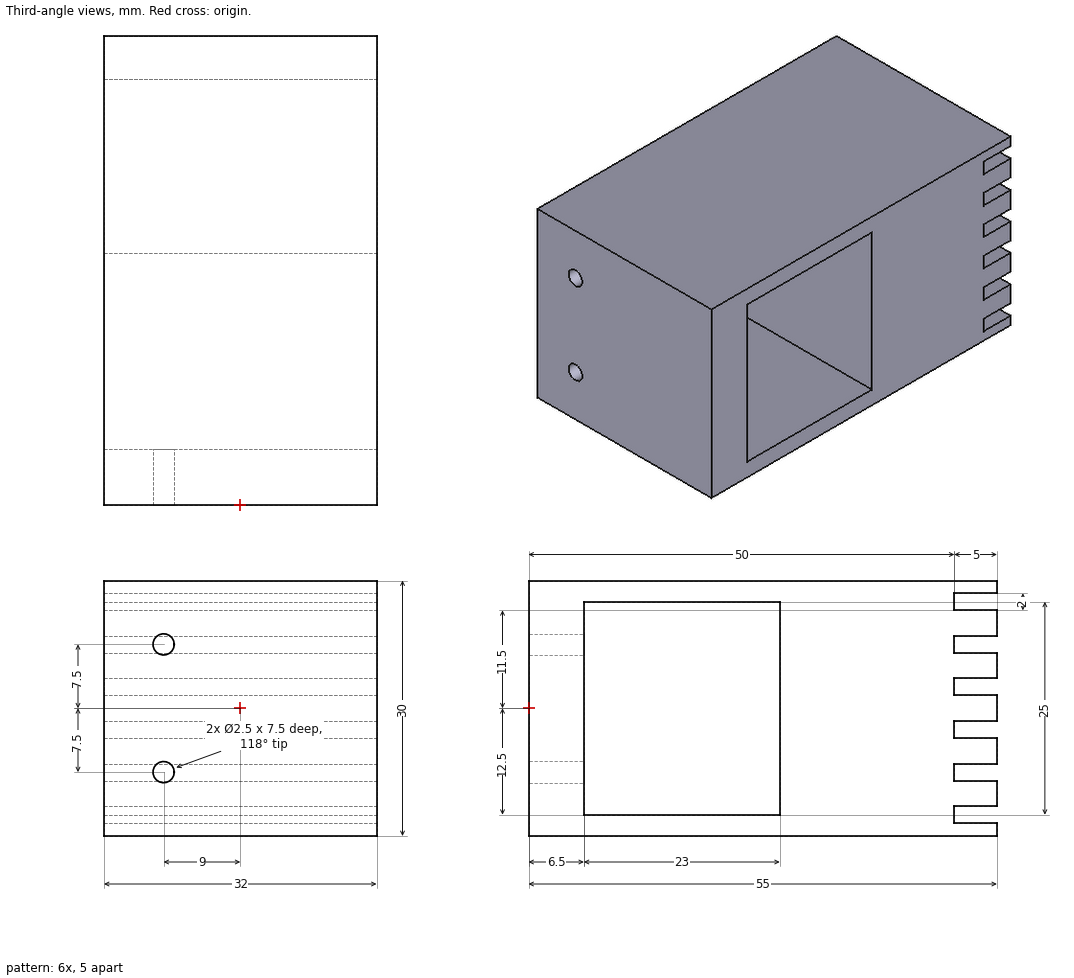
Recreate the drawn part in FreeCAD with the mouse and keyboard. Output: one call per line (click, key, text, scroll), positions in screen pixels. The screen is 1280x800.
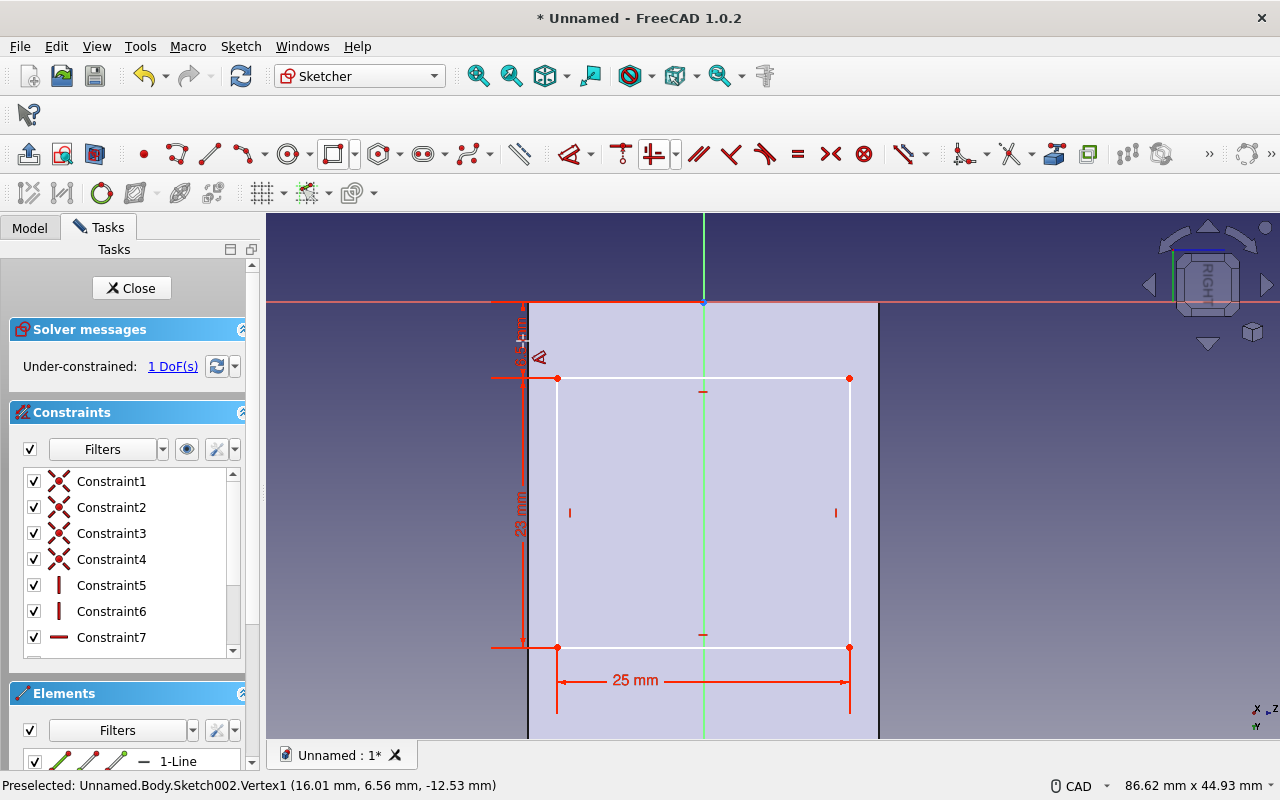
click(557, 378)
click(630, 268)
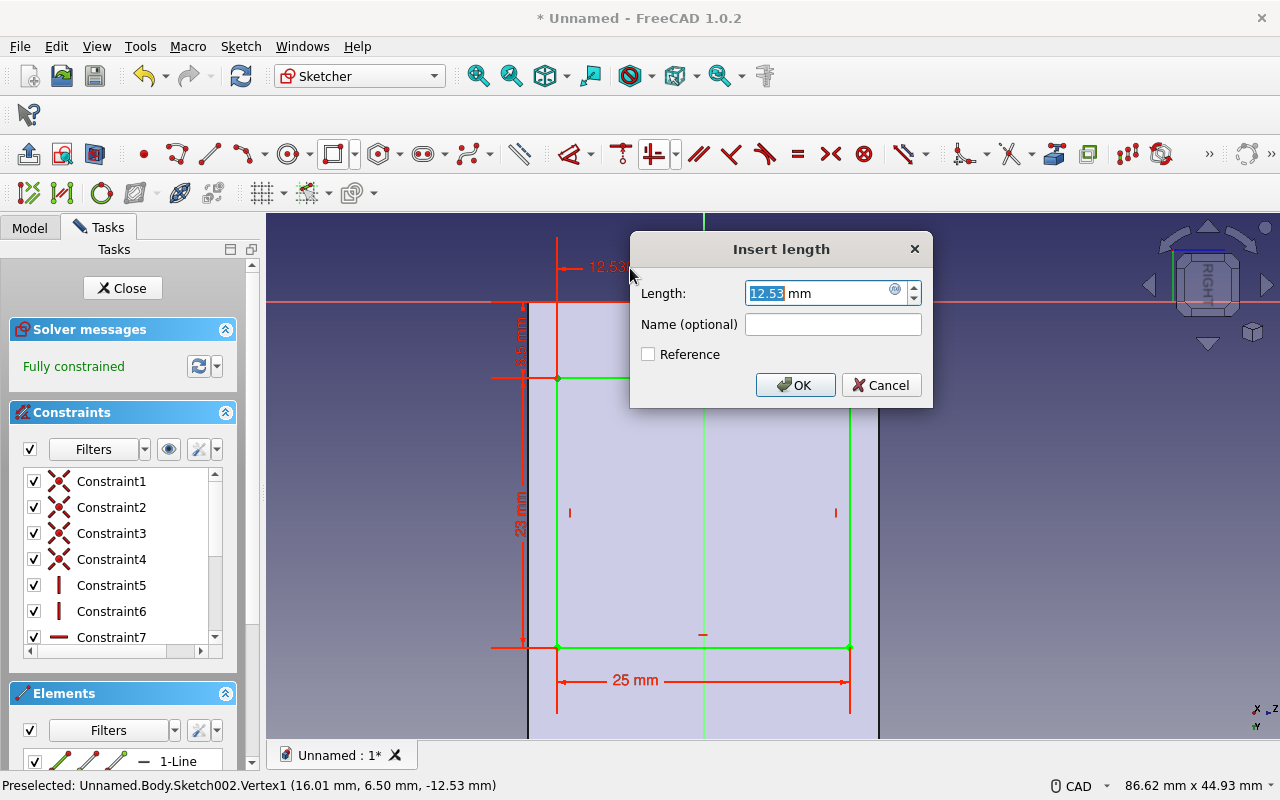
text(12.5)
key(Return)
key(Escape)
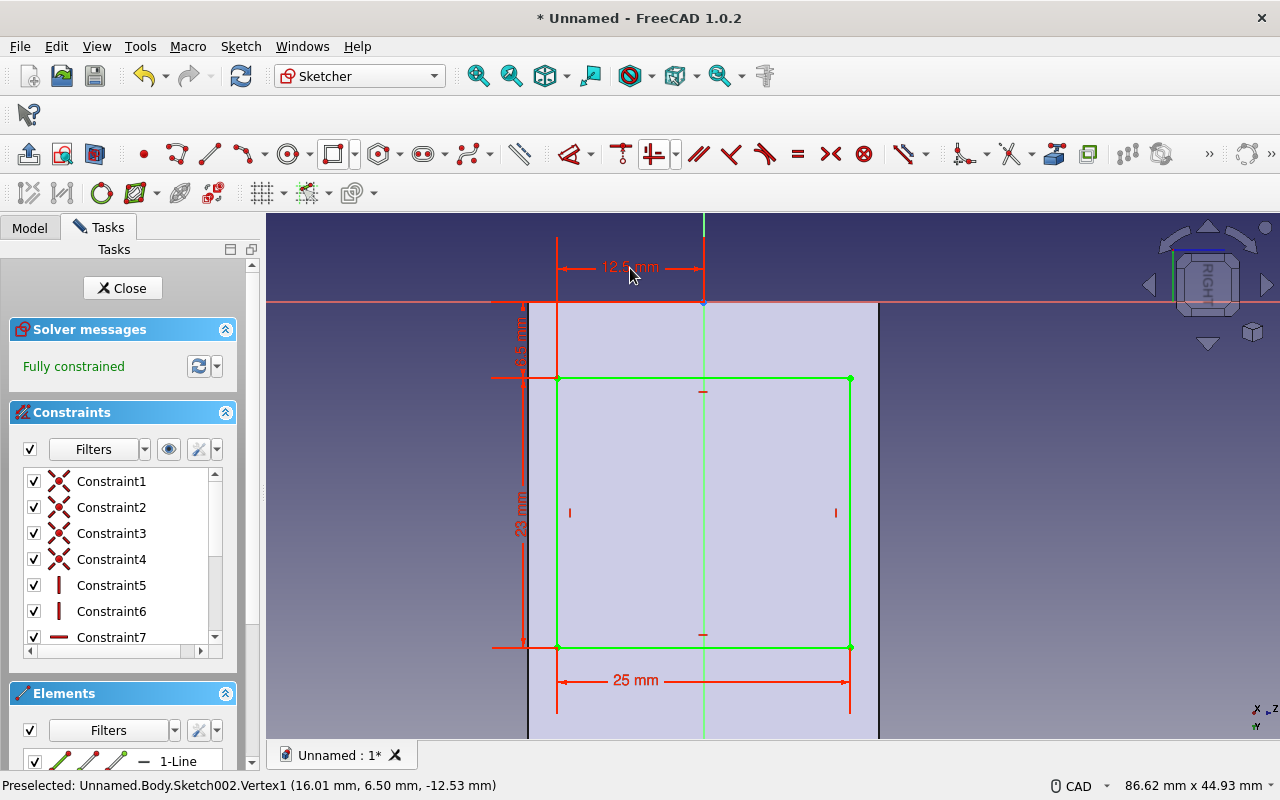
click(123, 288)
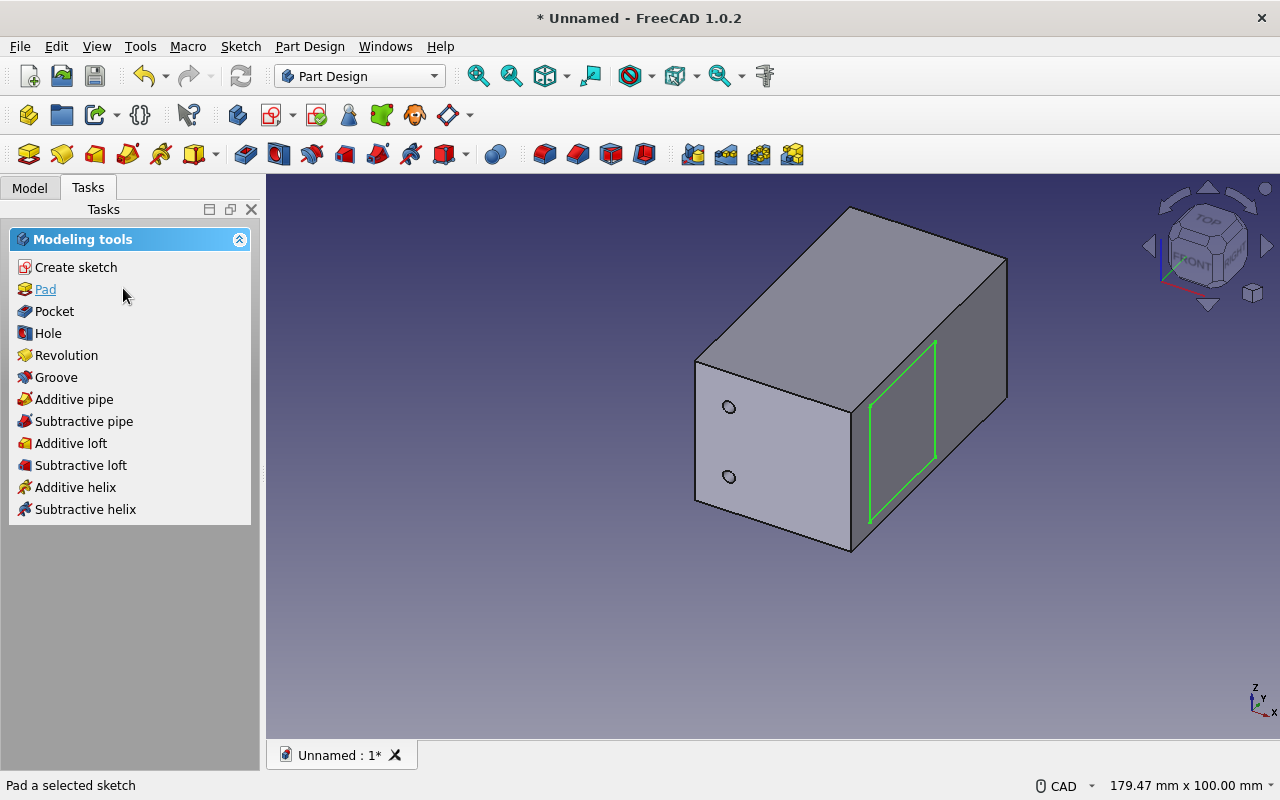
click(246, 154)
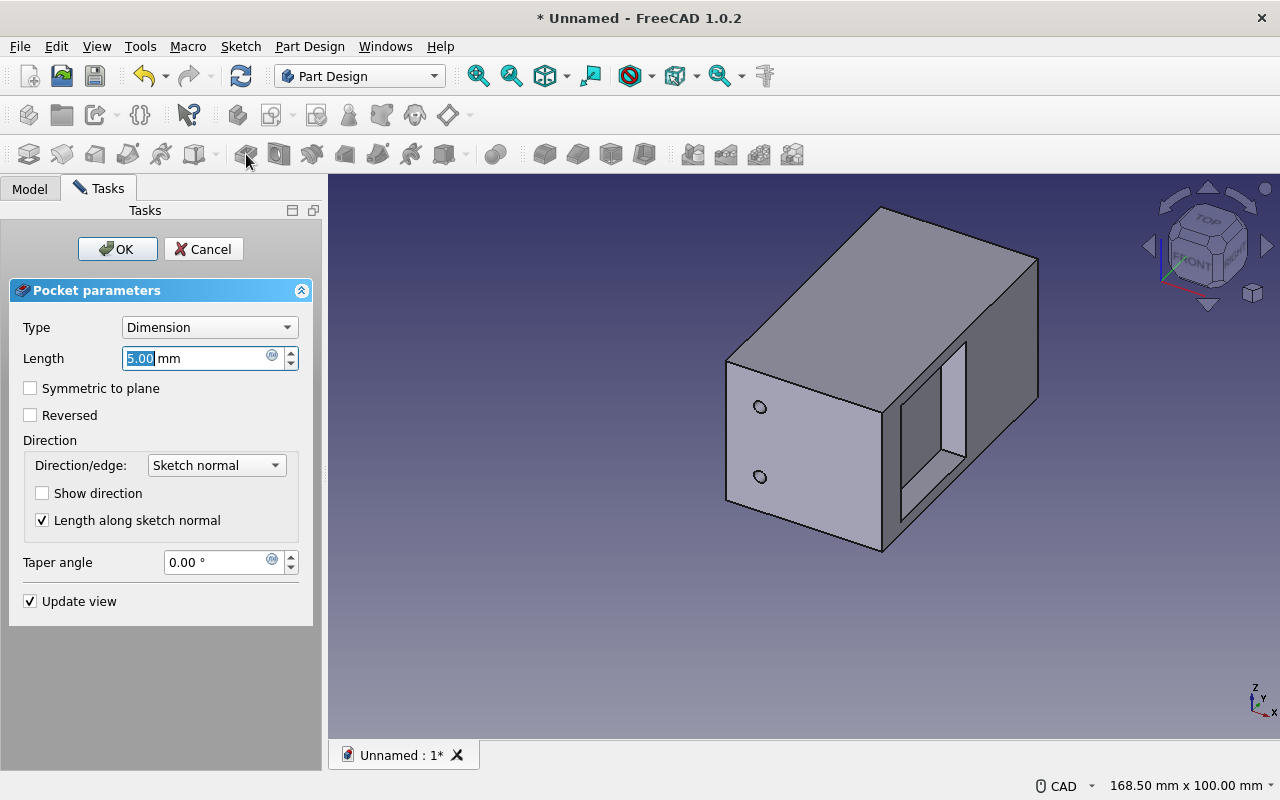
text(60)
key(Tab)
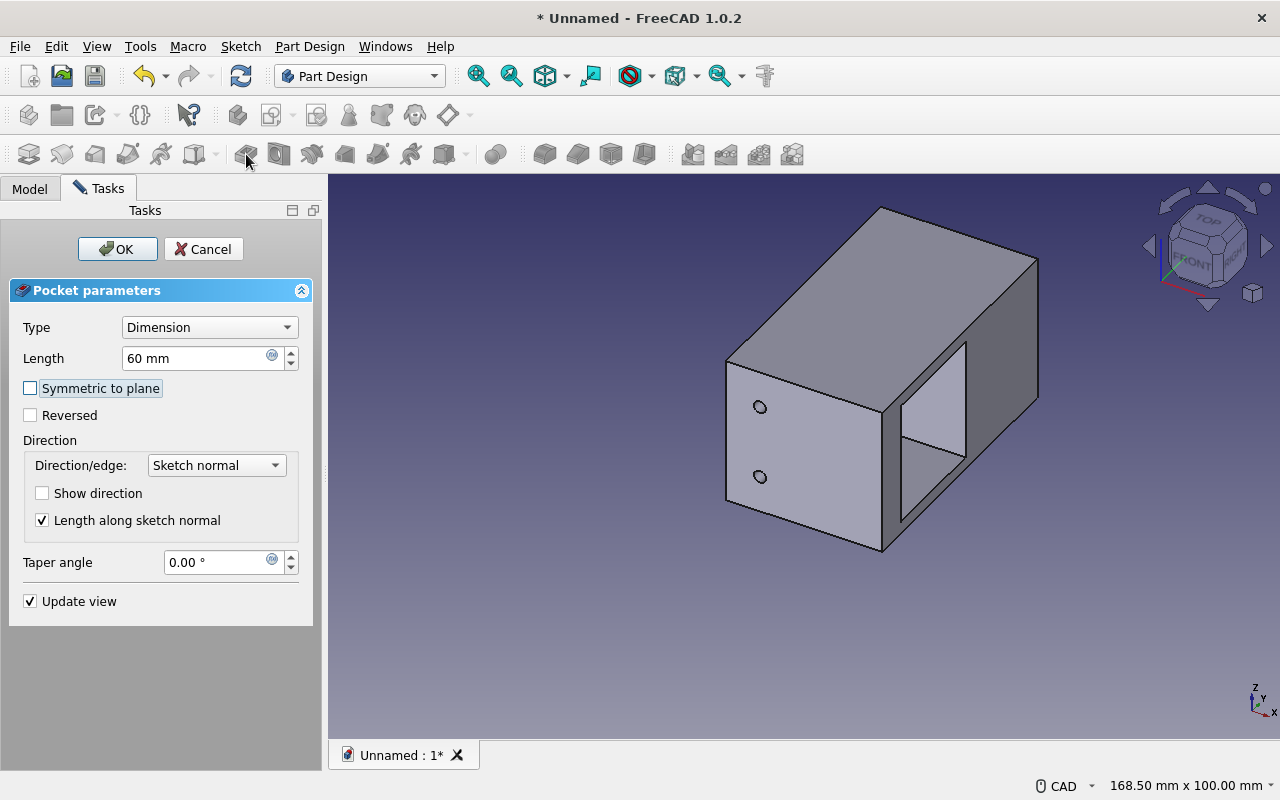
click(118, 249)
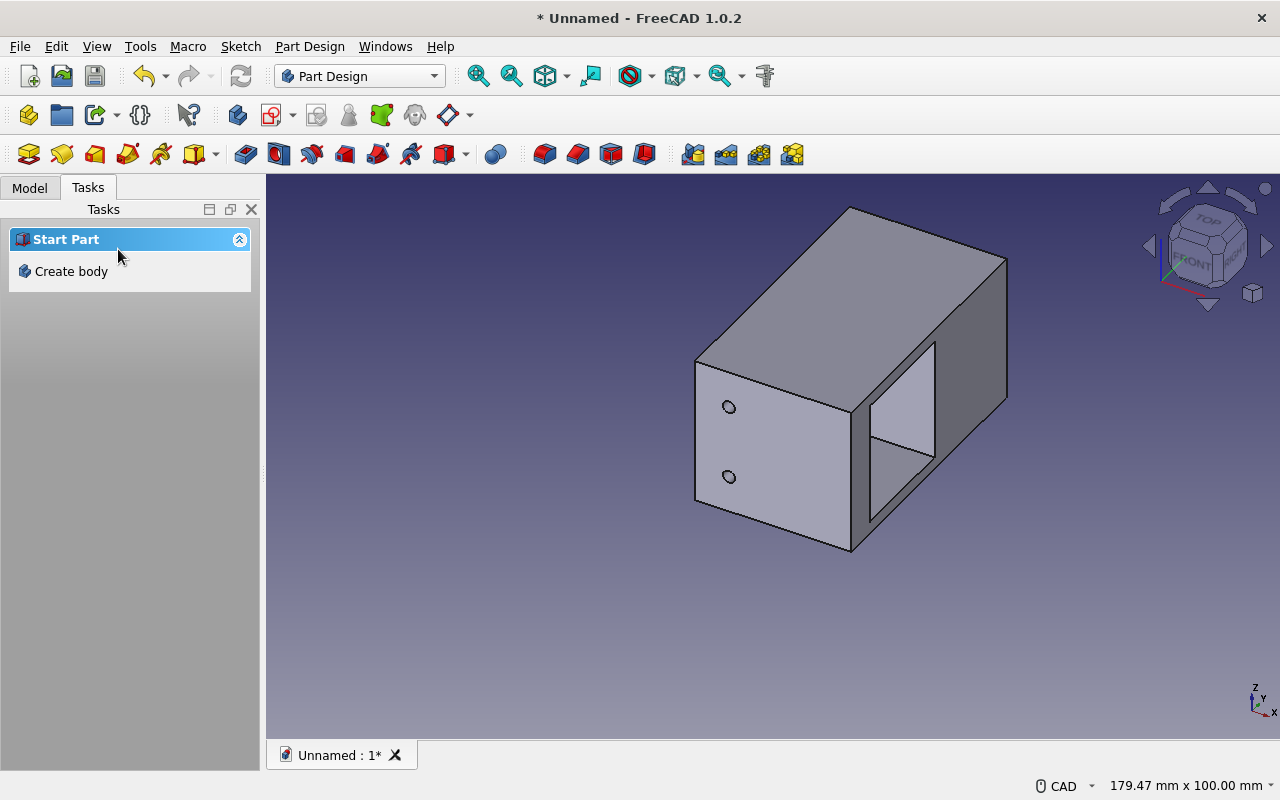
click(973, 360)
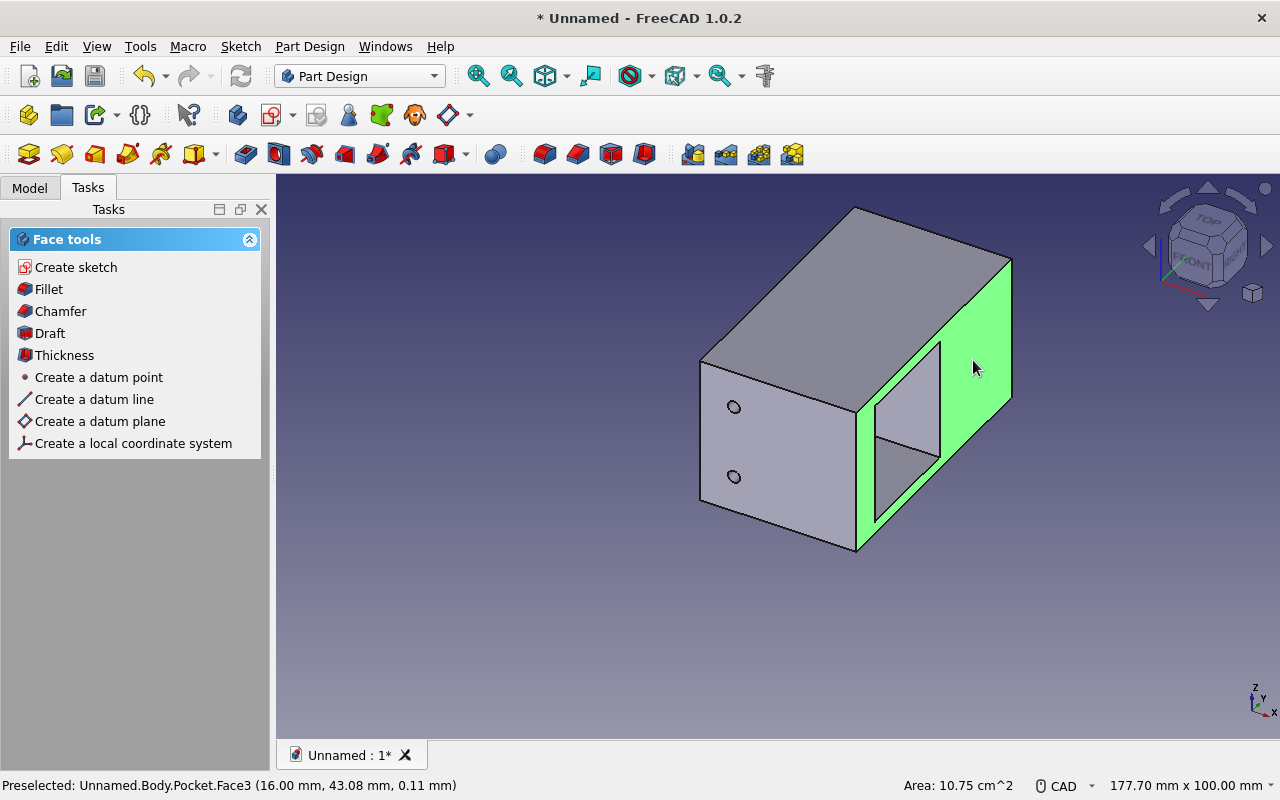
click(270, 116)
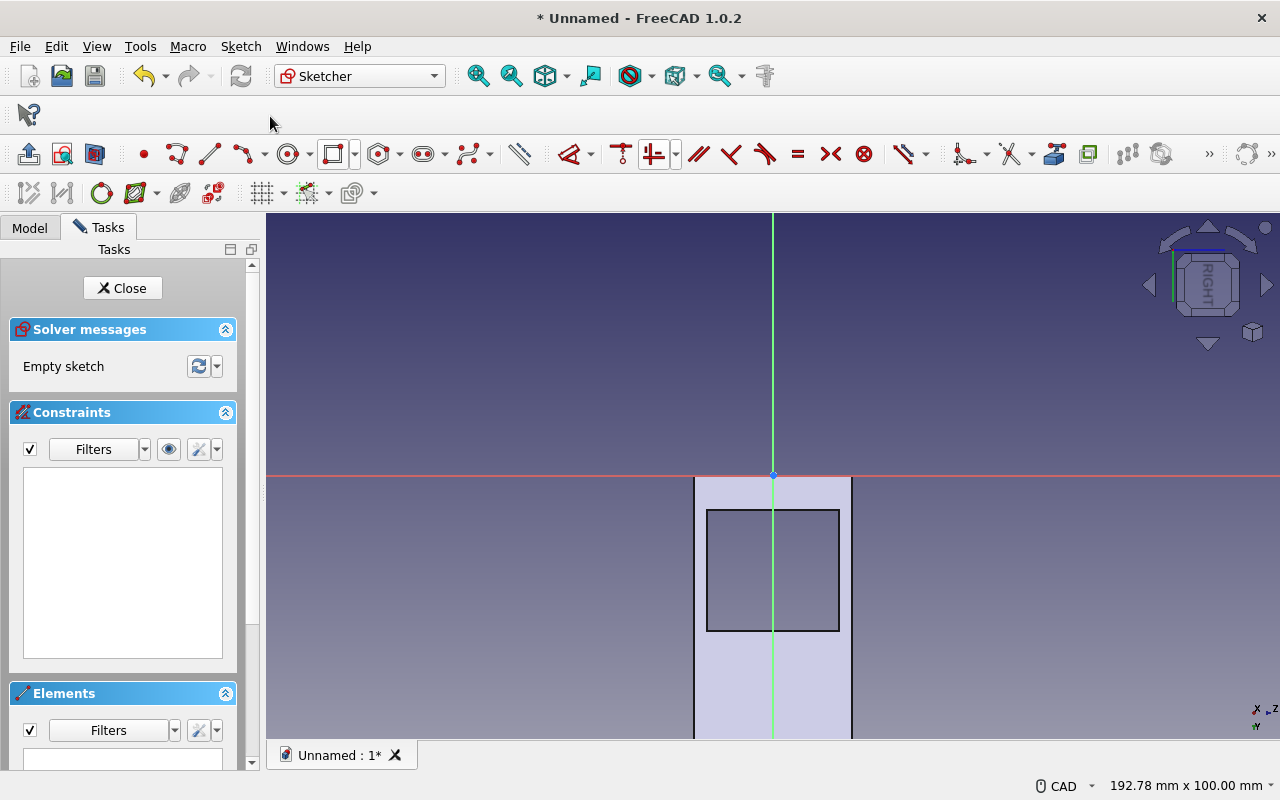
scroll(704, 476, down, 5)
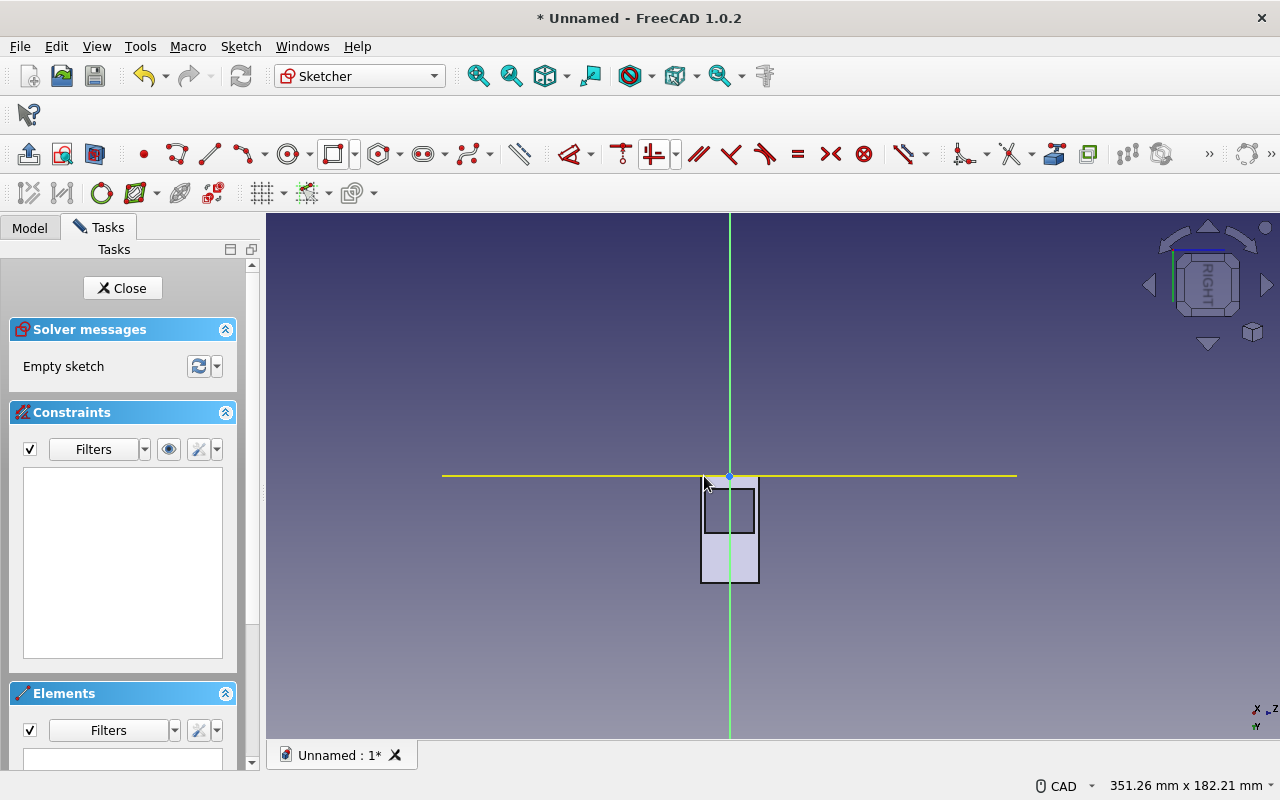
scroll(756, 583, up, 15)